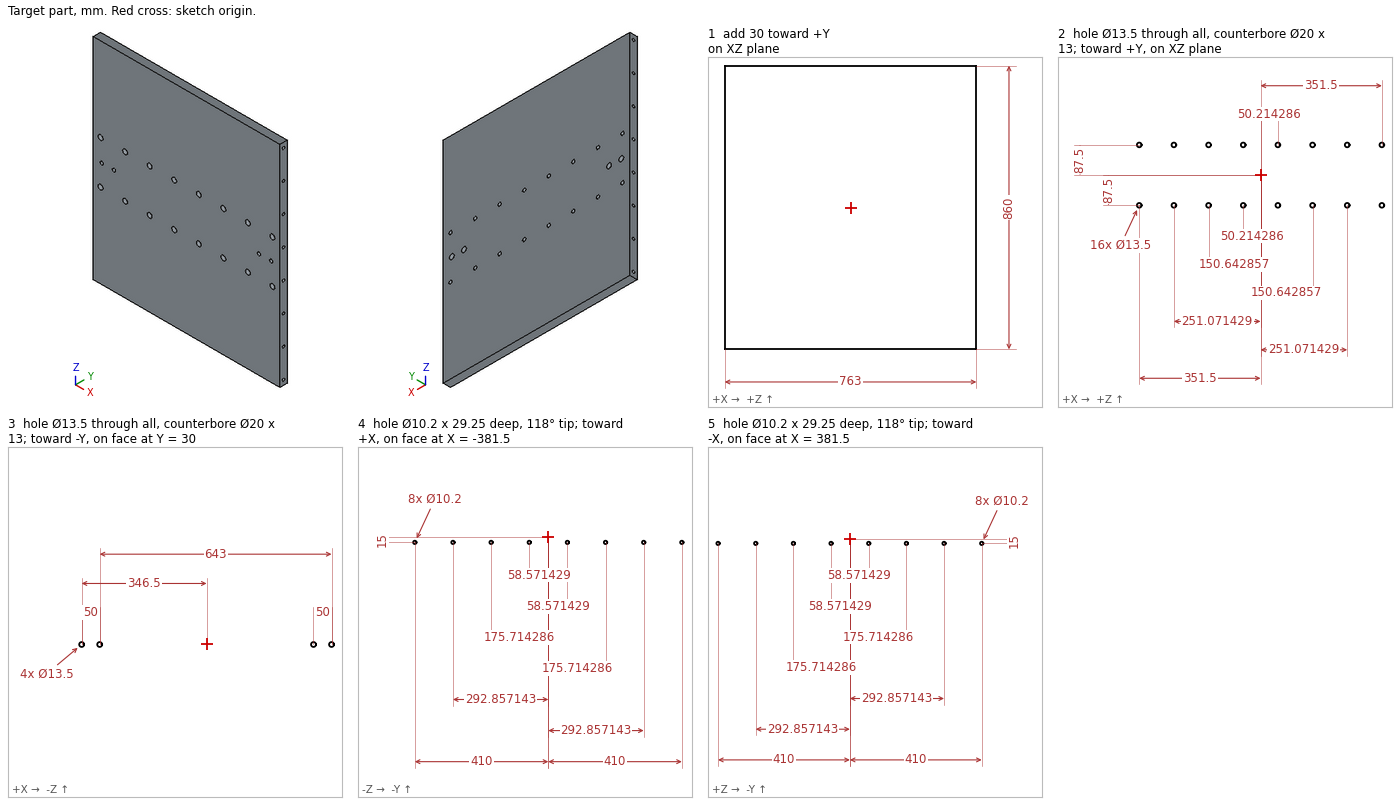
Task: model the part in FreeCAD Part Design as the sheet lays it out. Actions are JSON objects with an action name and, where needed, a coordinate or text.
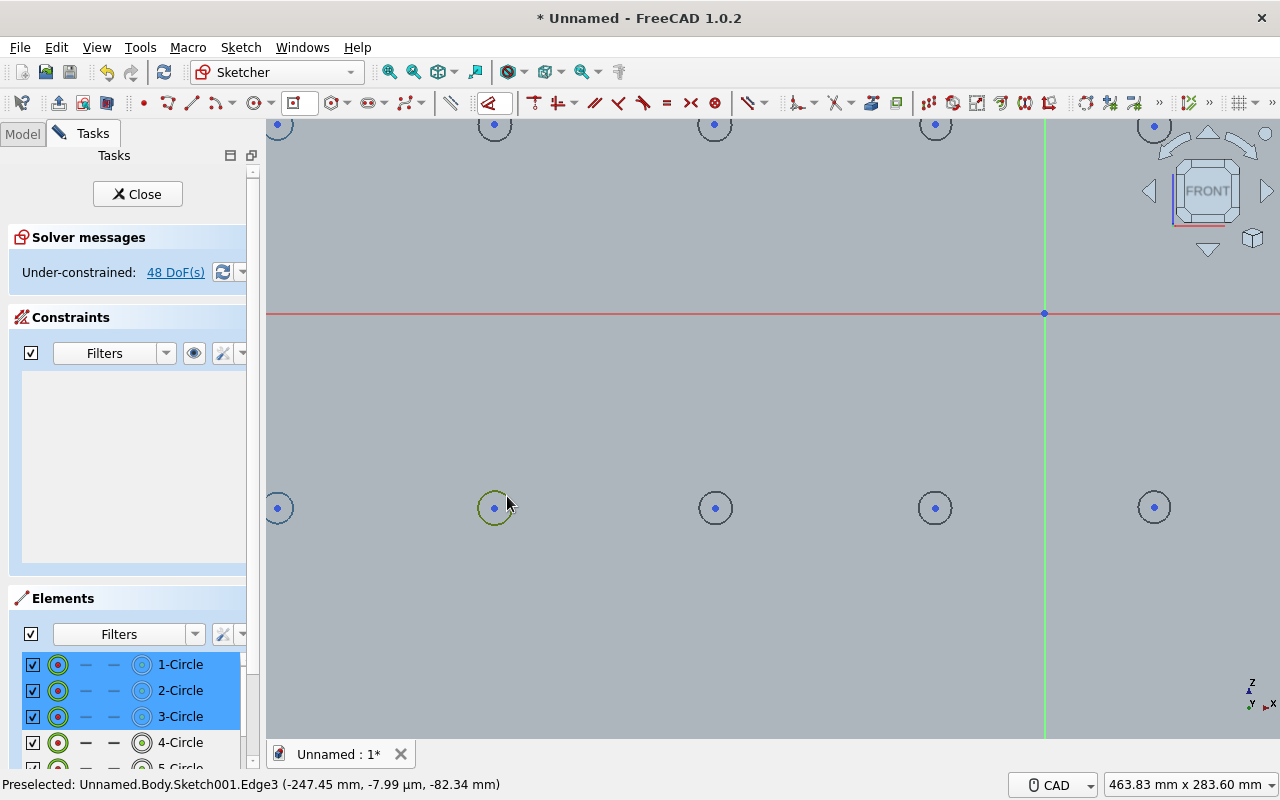
{"action": "scroll", "coordinate": [506, 496], "scroll_direction": "down", "scroll_amount": 5}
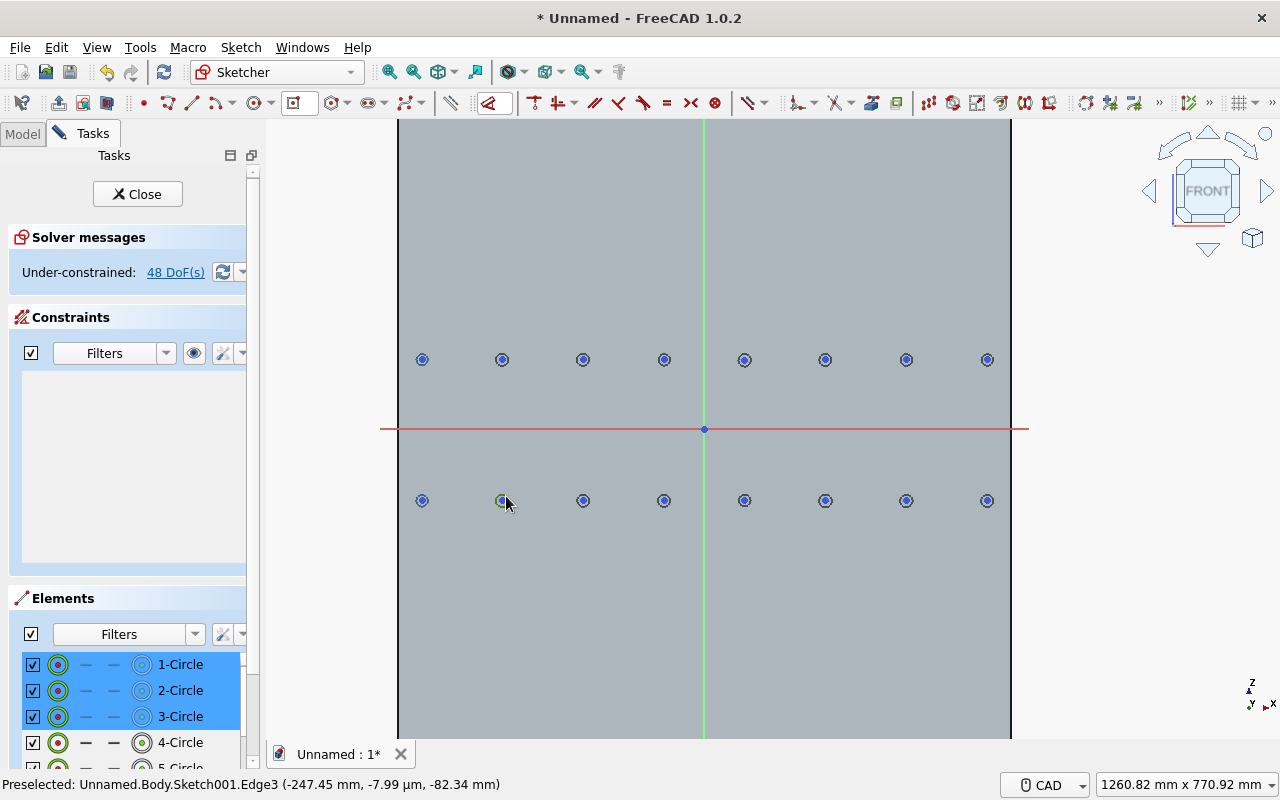
{"action": "scroll", "coordinate": [506, 355], "scroll_direction": "up", "scroll_amount": 5}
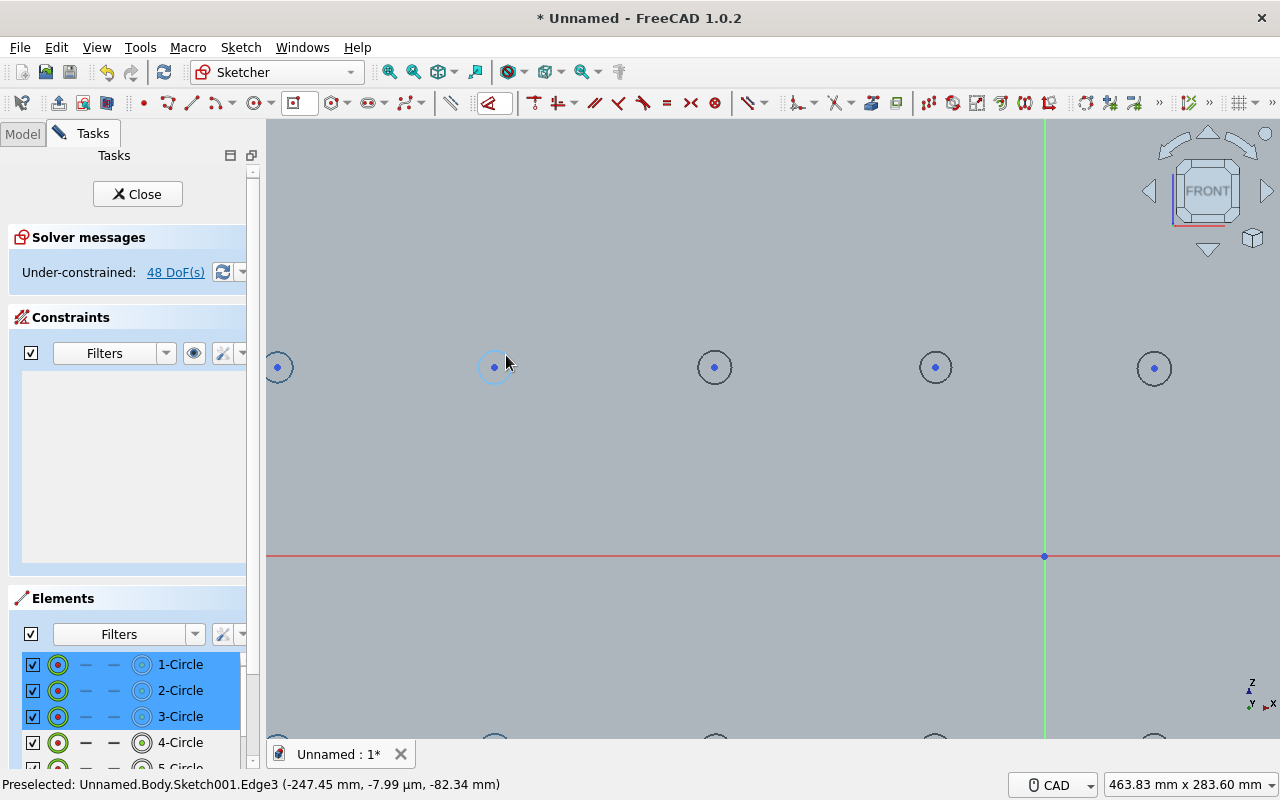
{"action": "left_click", "coordinate": [507, 356]}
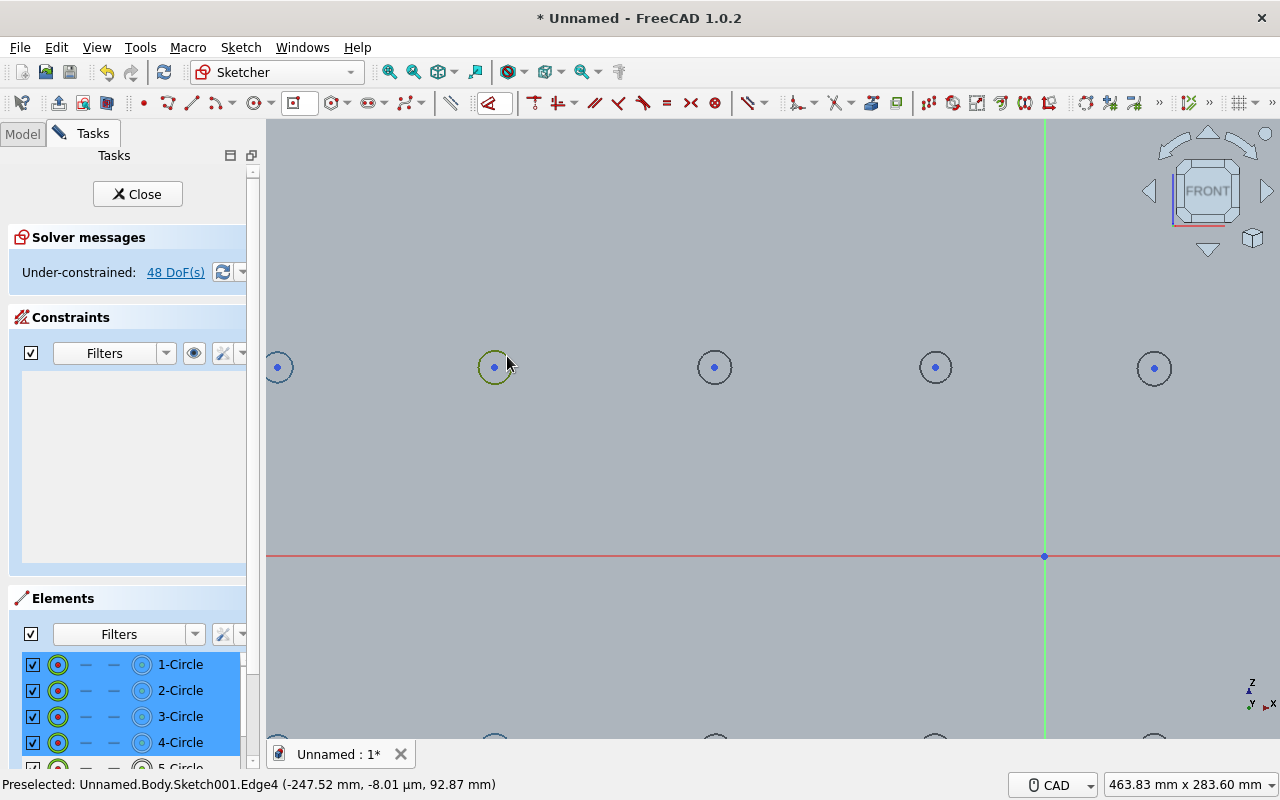
{"action": "scroll", "coordinate": [506, 355], "scroll_direction": "down", "scroll_amount": 5}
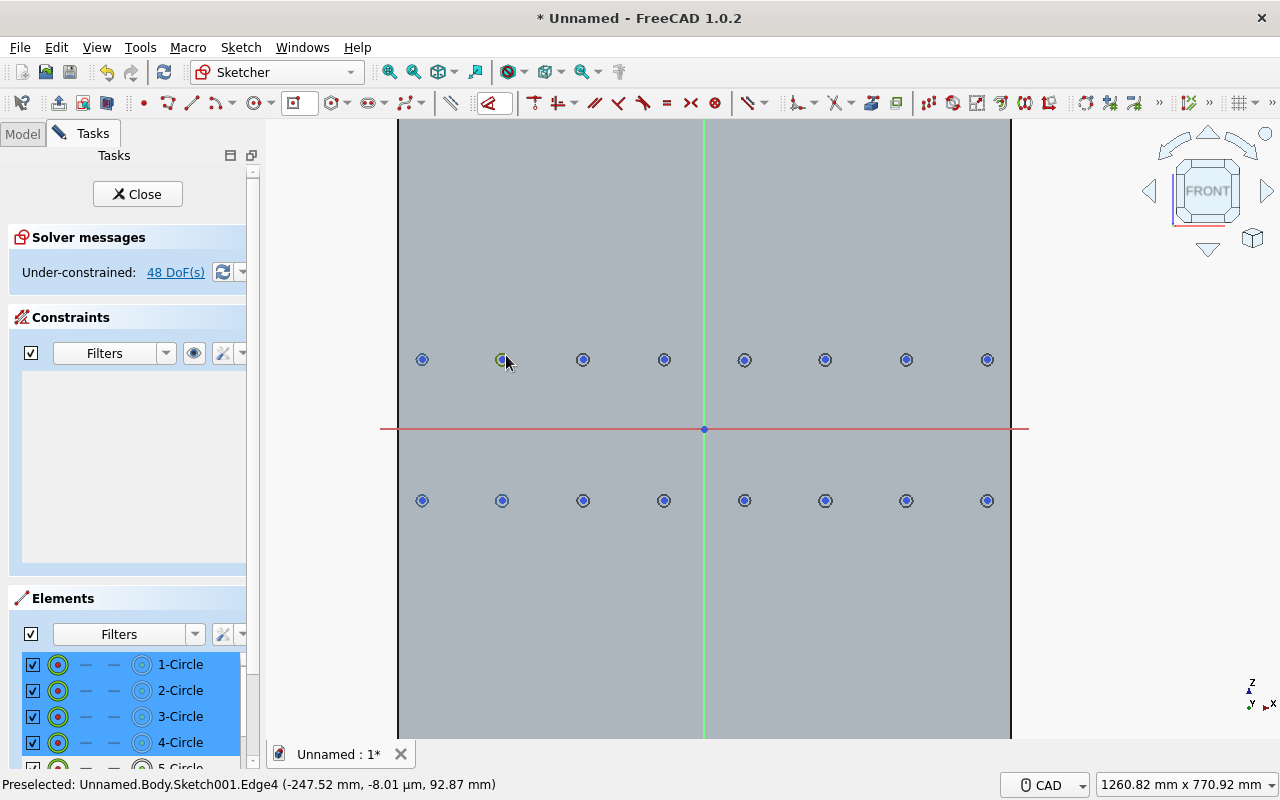
{"action": "scroll", "coordinate": [588, 497], "scroll_direction": "up", "scroll_amount": 5}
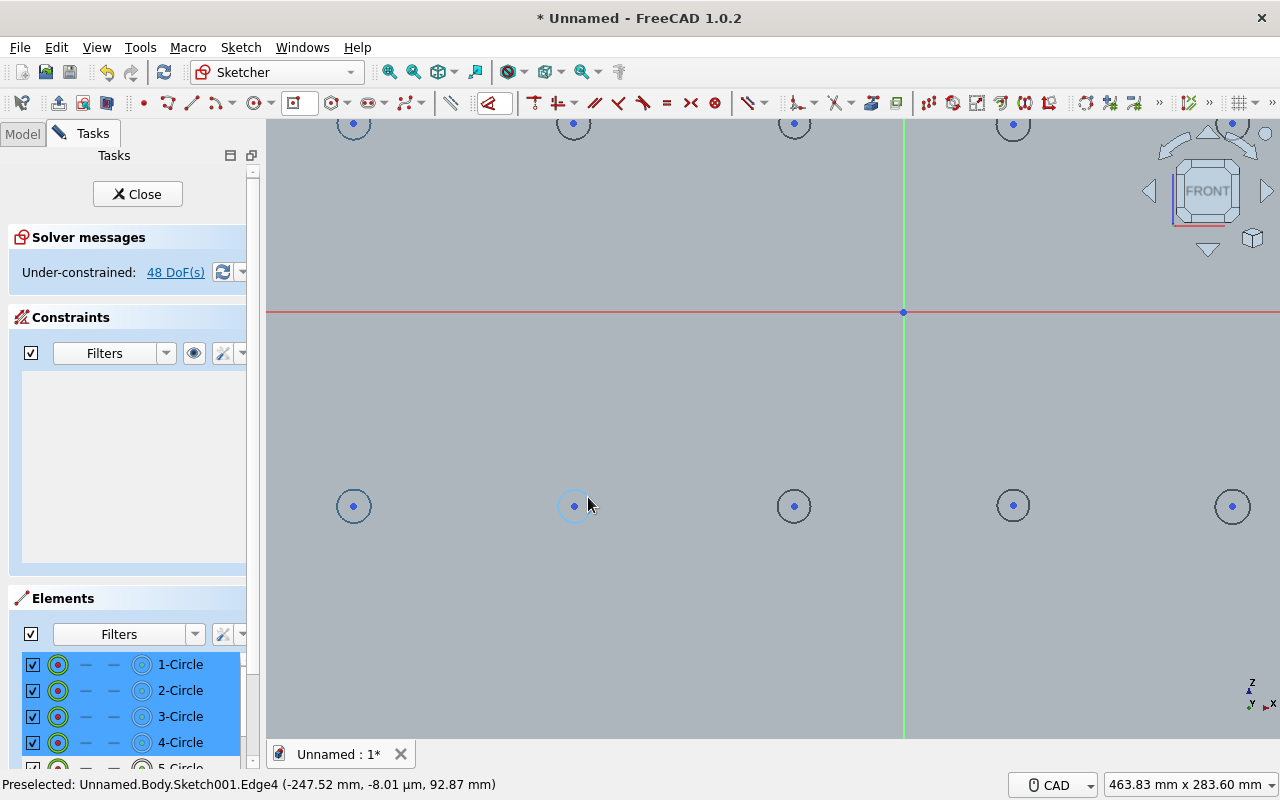
{"action": "left_click", "coordinate": [586, 495]}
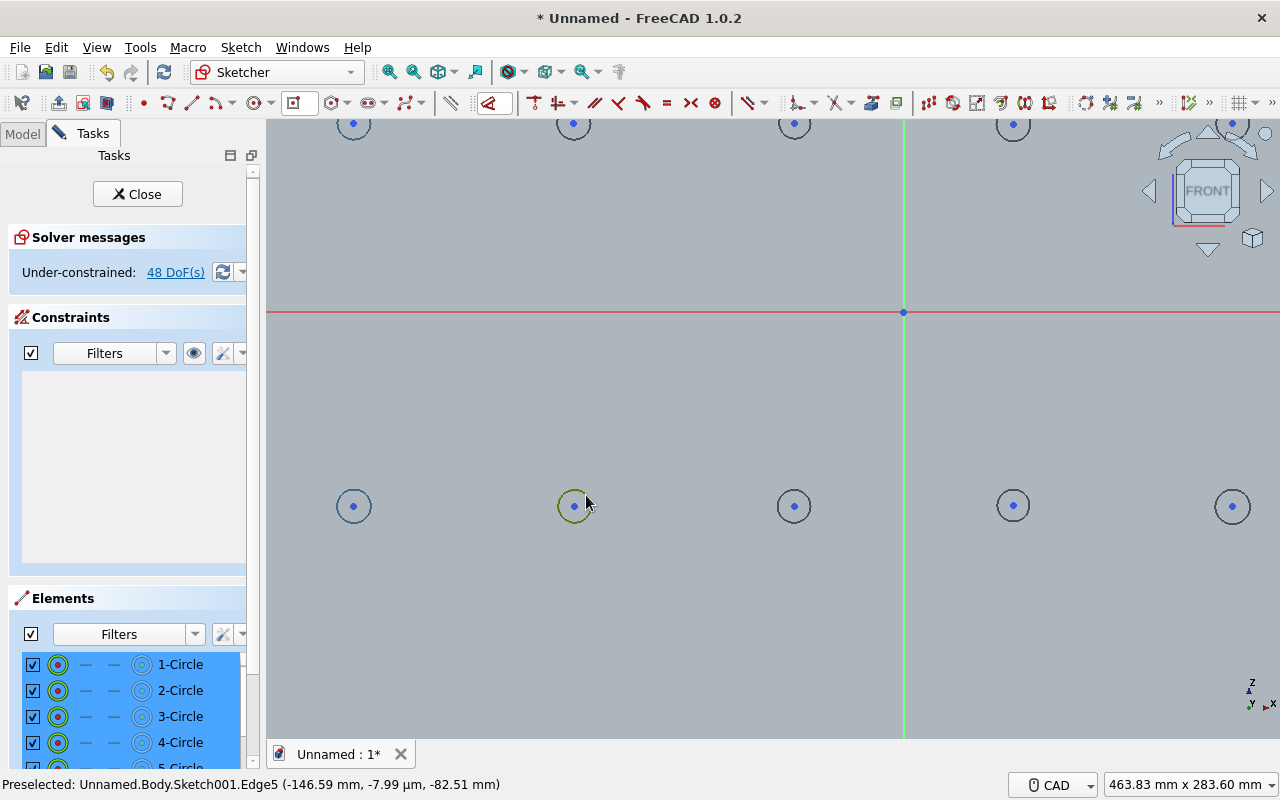
{"action": "scroll", "coordinate": [588, 497], "scroll_direction": "down", "scroll_amount": 5}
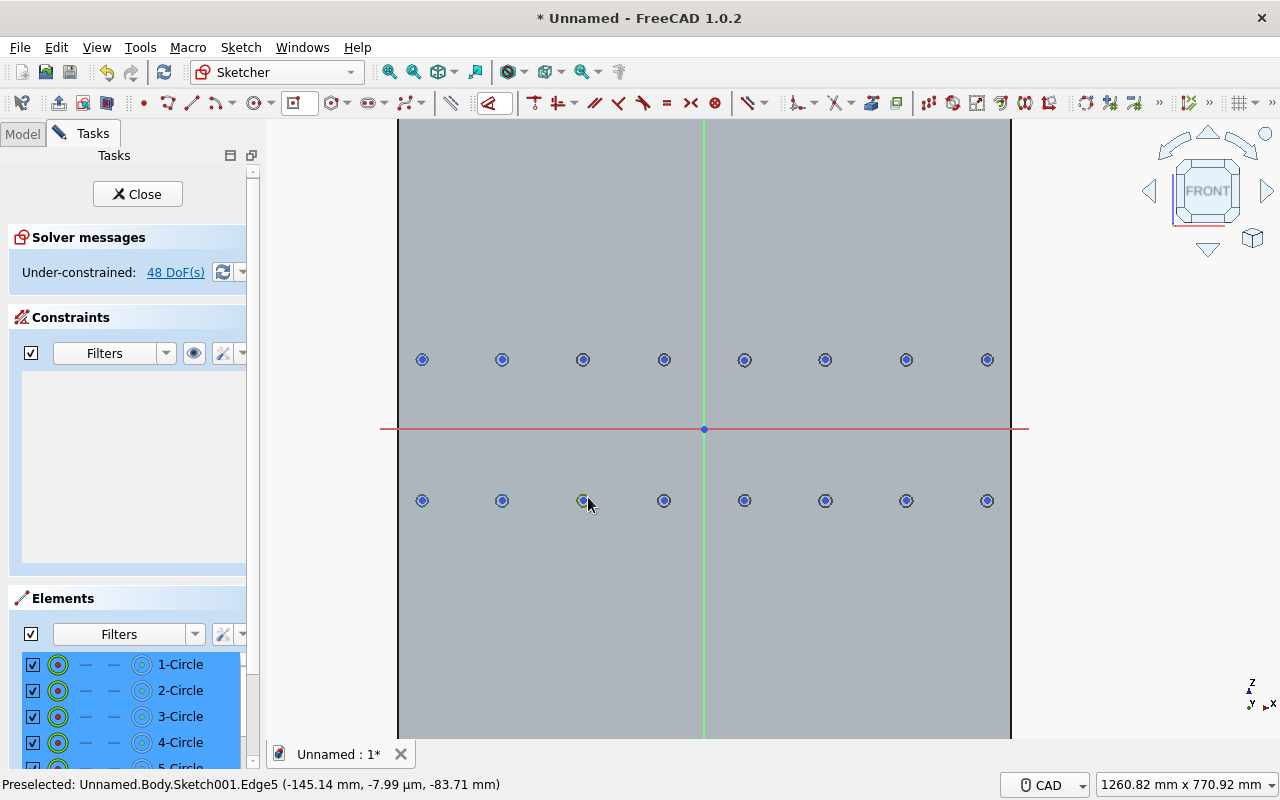
{"action": "scroll", "coordinate": [587, 355], "scroll_direction": "up", "scroll_amount": 5}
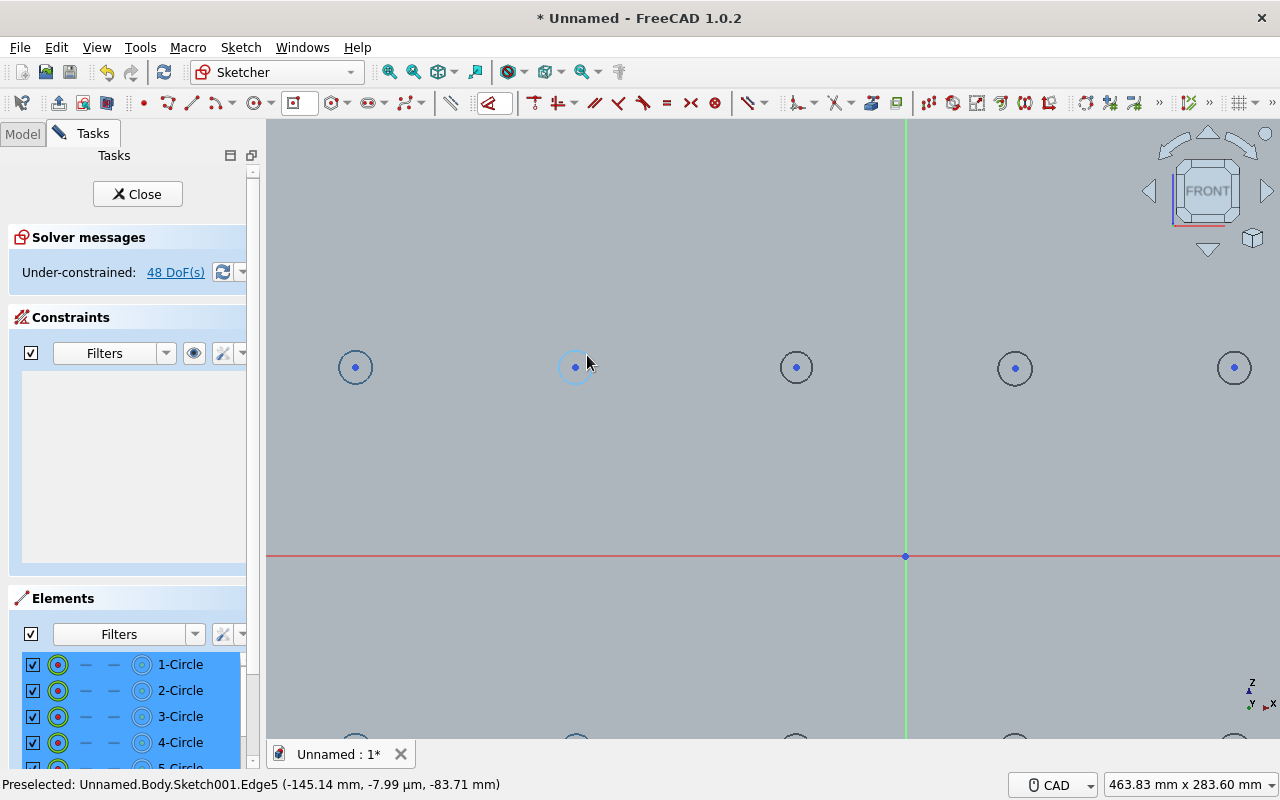
{"action": "left_click", "coordinate": [587, 356]}